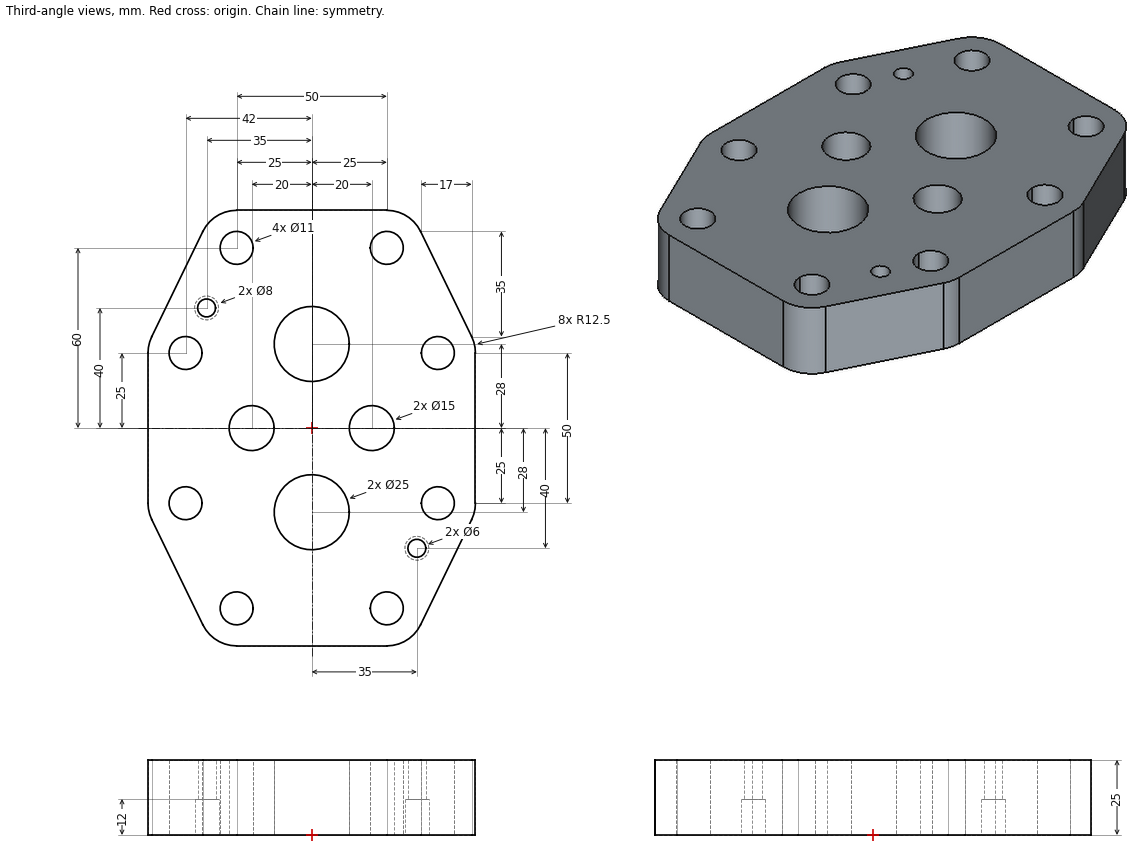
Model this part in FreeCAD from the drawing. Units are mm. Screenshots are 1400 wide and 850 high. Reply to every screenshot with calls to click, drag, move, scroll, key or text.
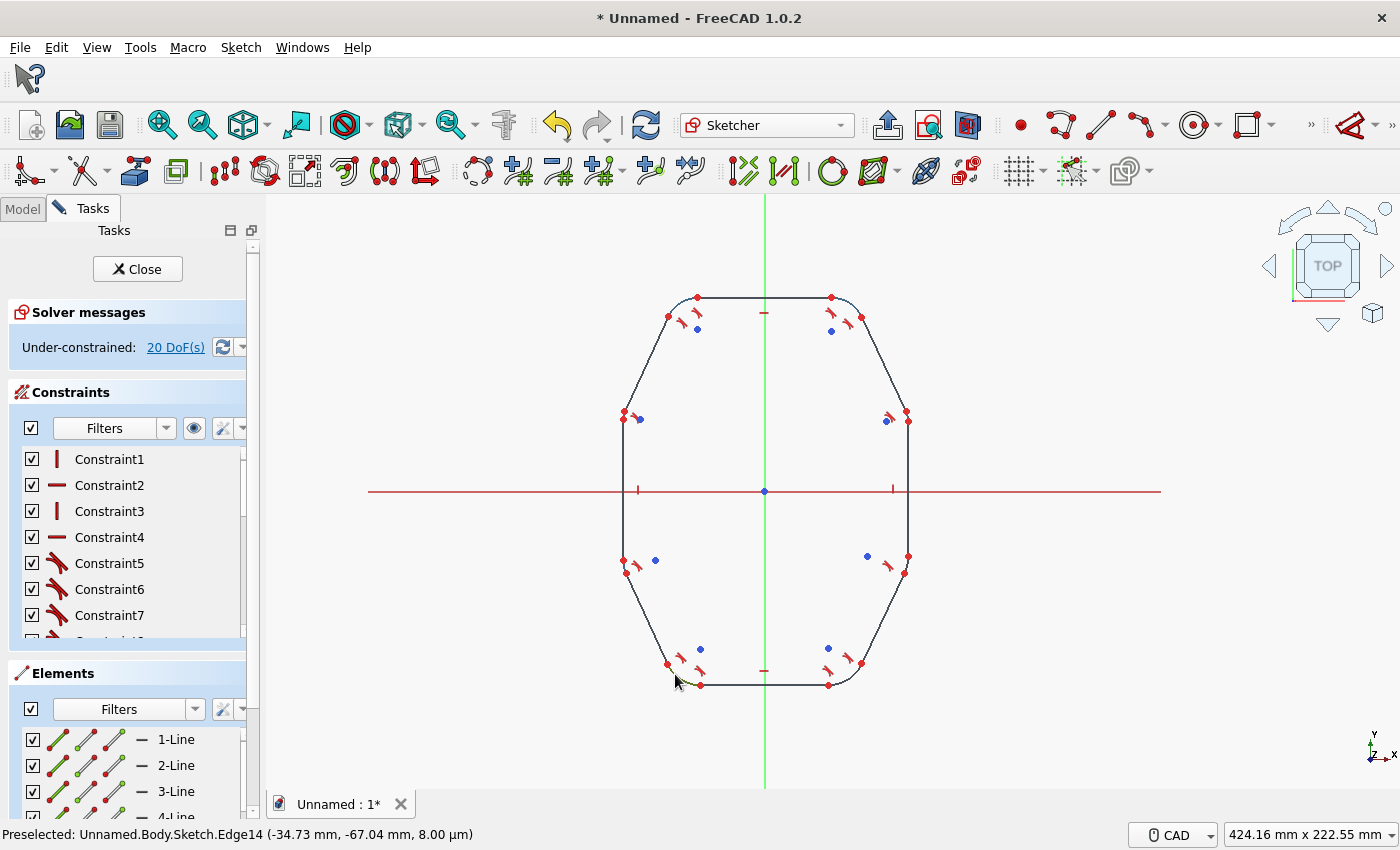
click(841, 683)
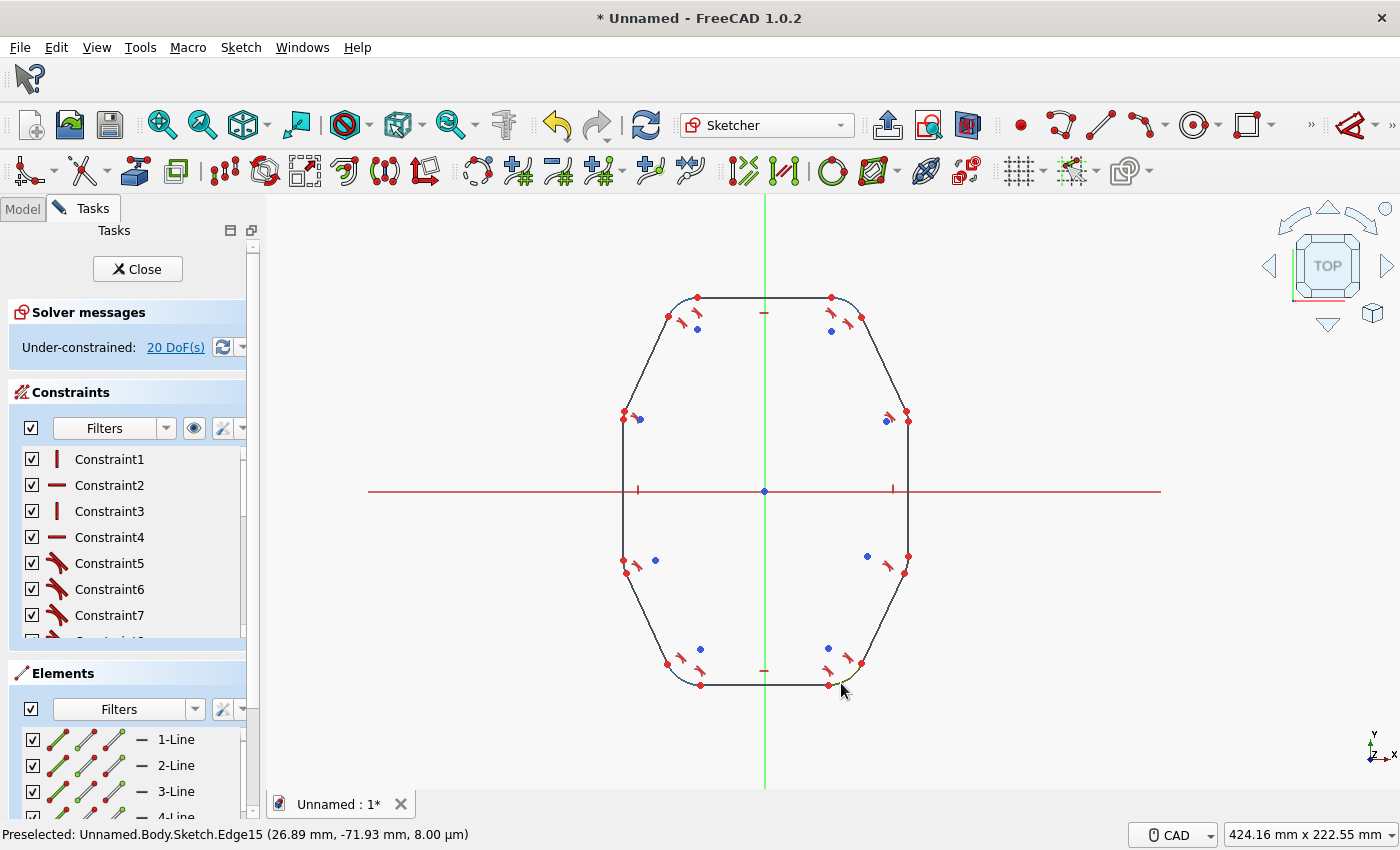
scroll(907, 565, up, 3)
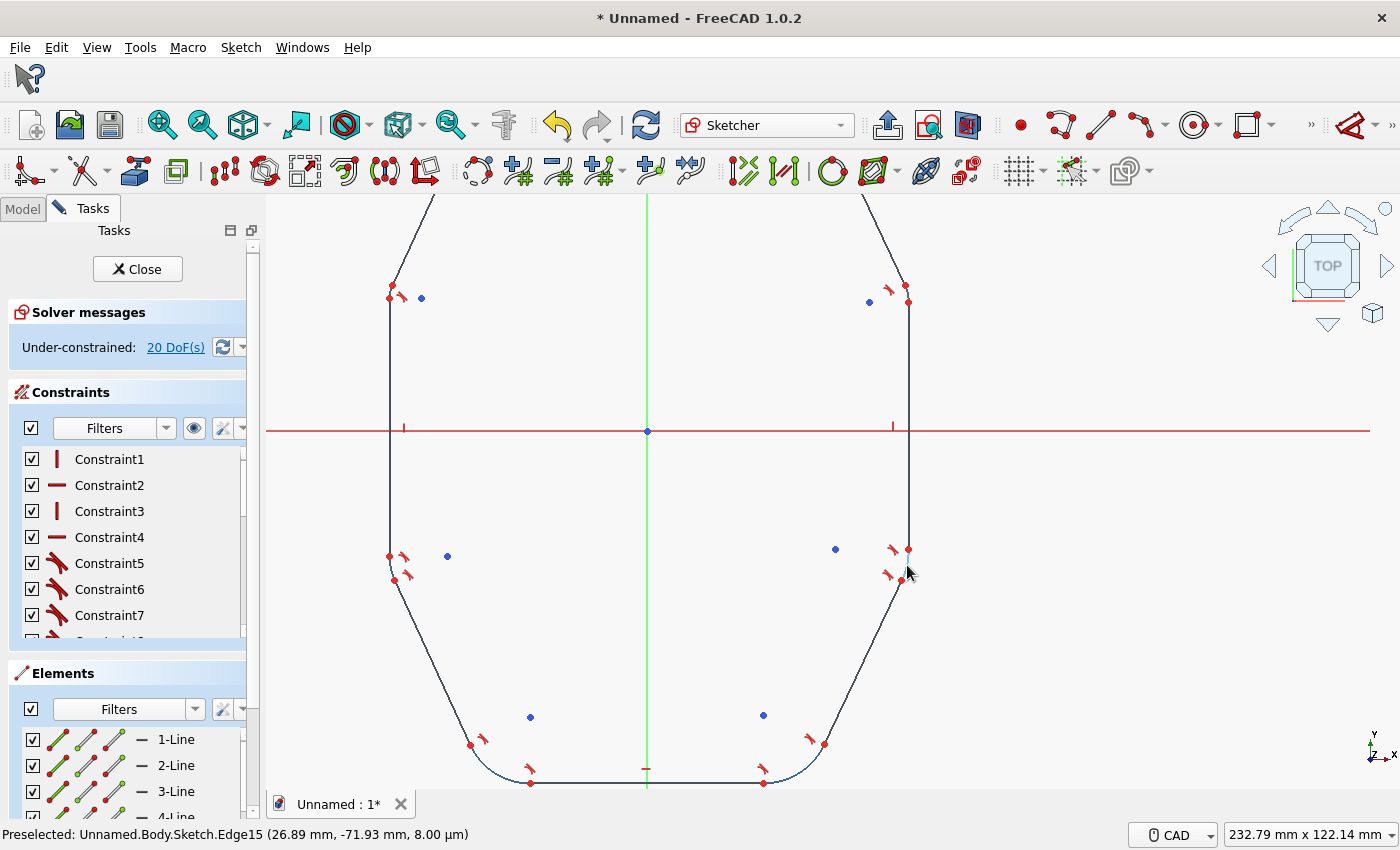
click(907, 565)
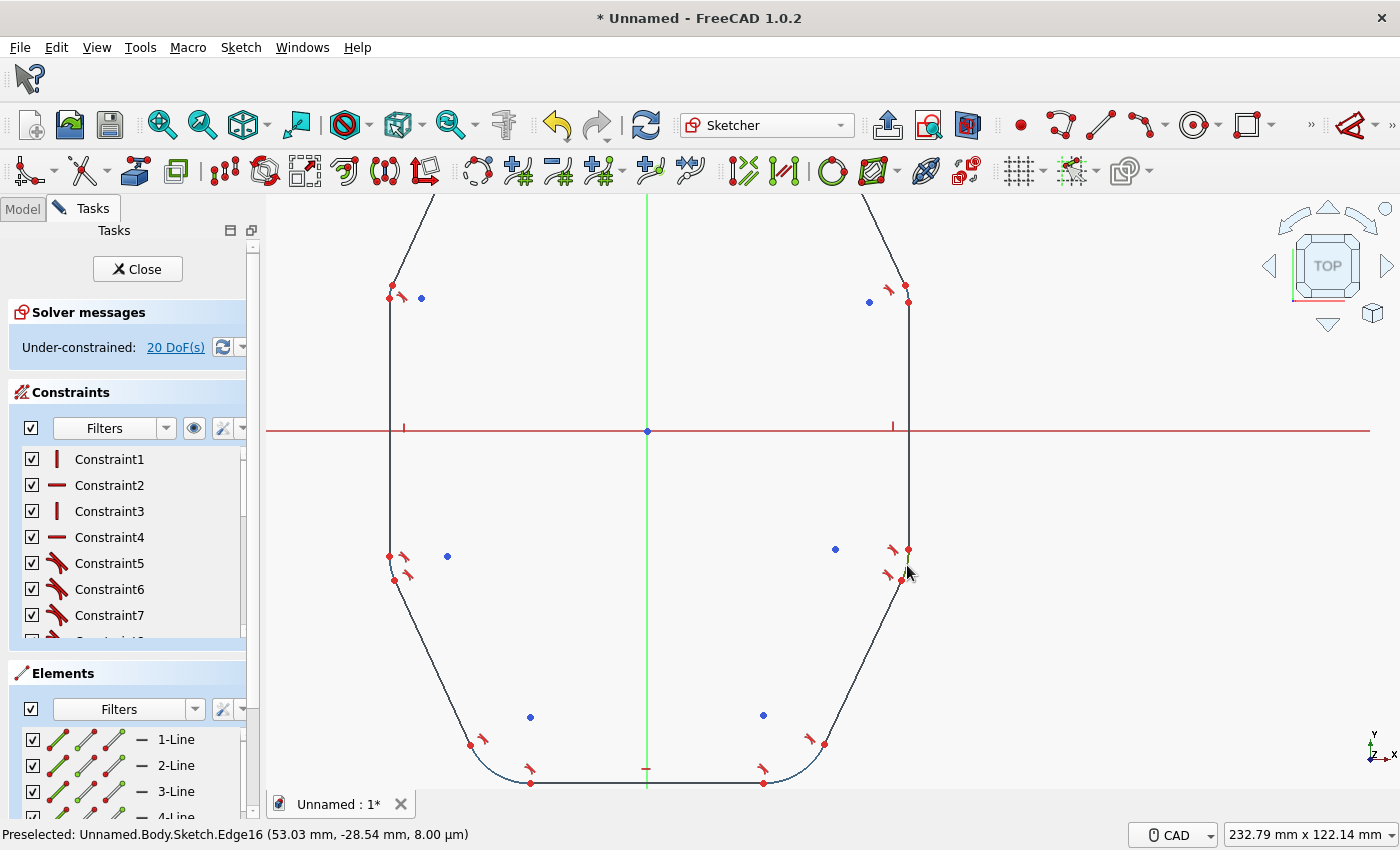
key(e)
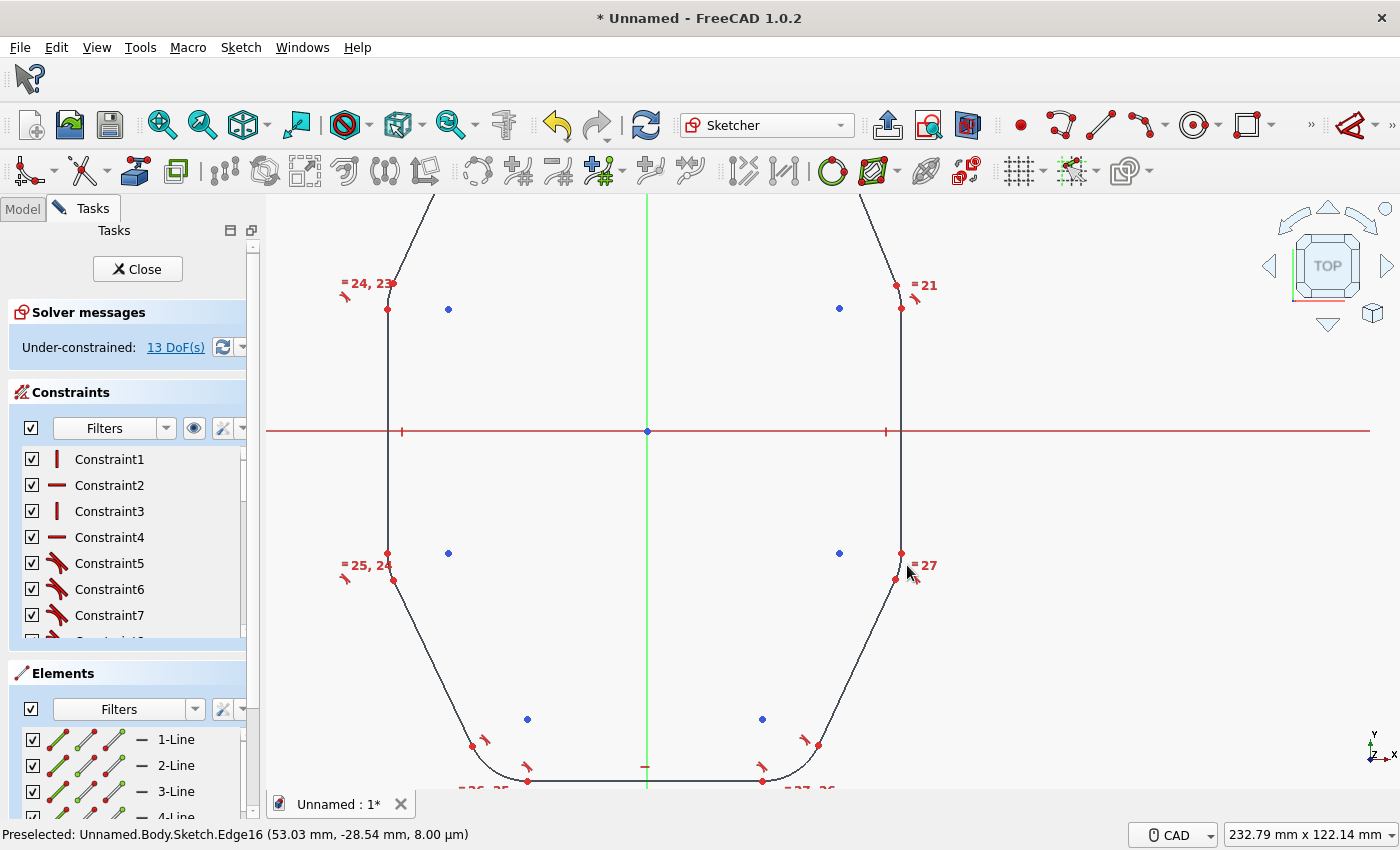
click(840, 308)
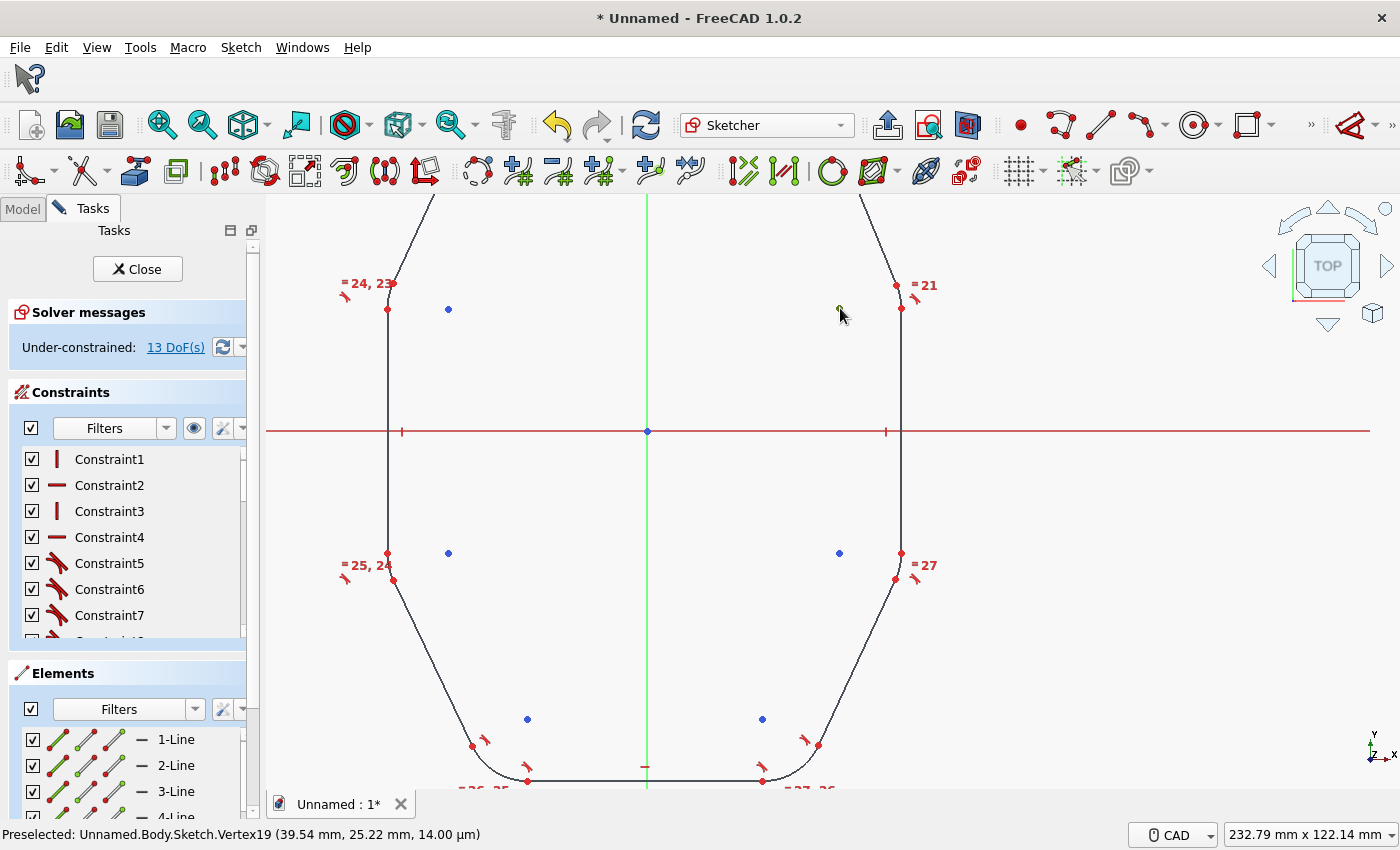
click(449, 309)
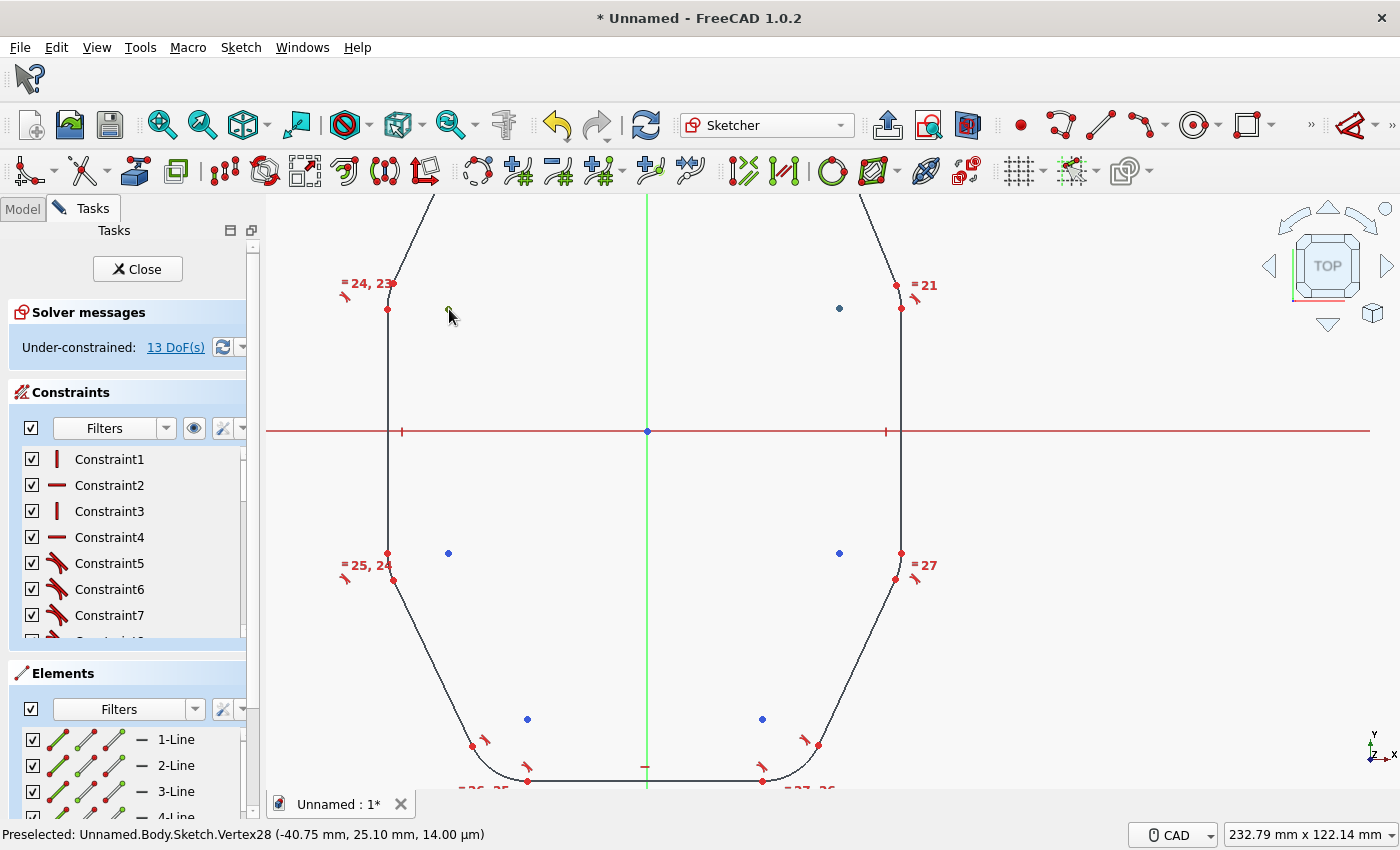
click(647, 722)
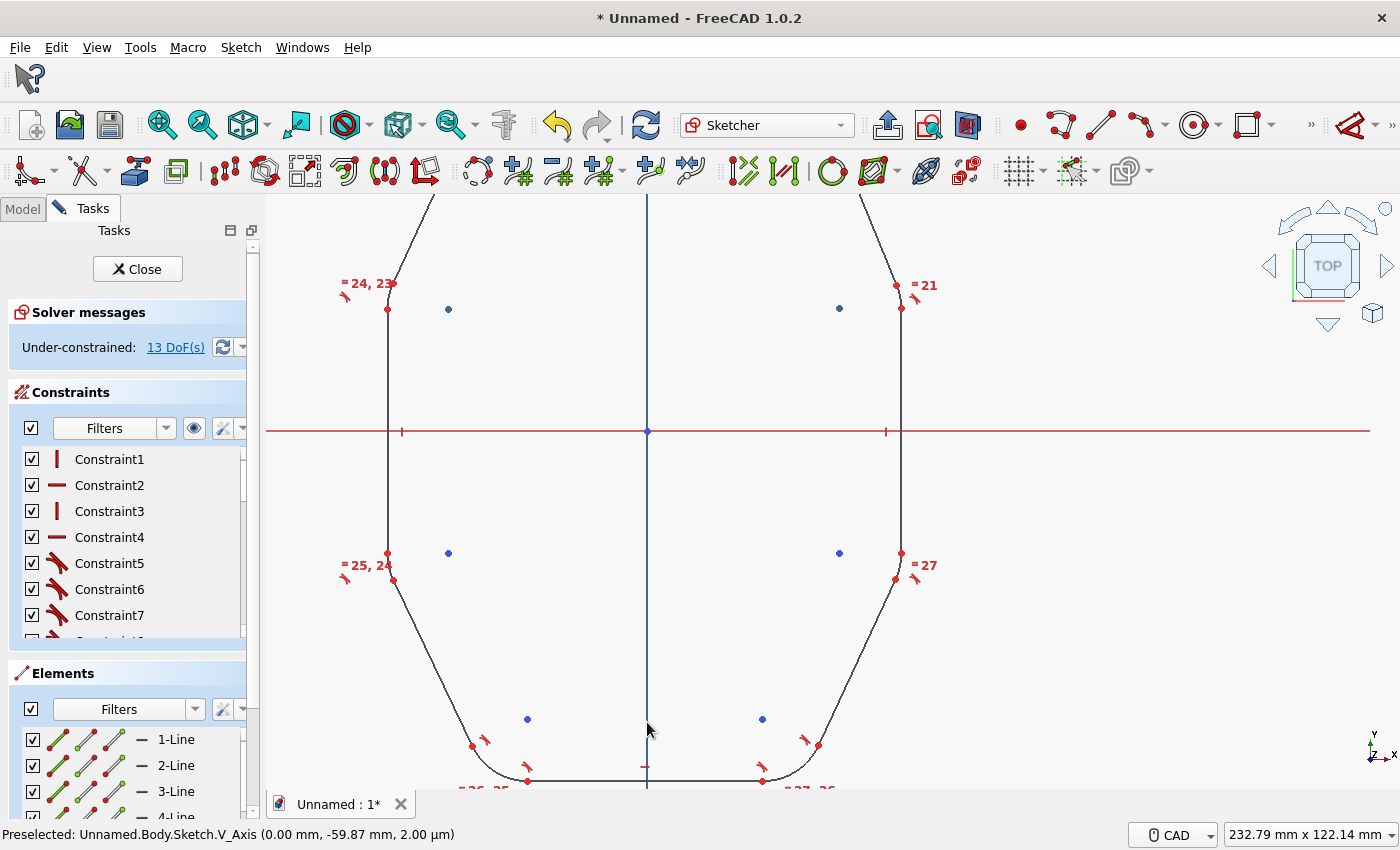
key(s)